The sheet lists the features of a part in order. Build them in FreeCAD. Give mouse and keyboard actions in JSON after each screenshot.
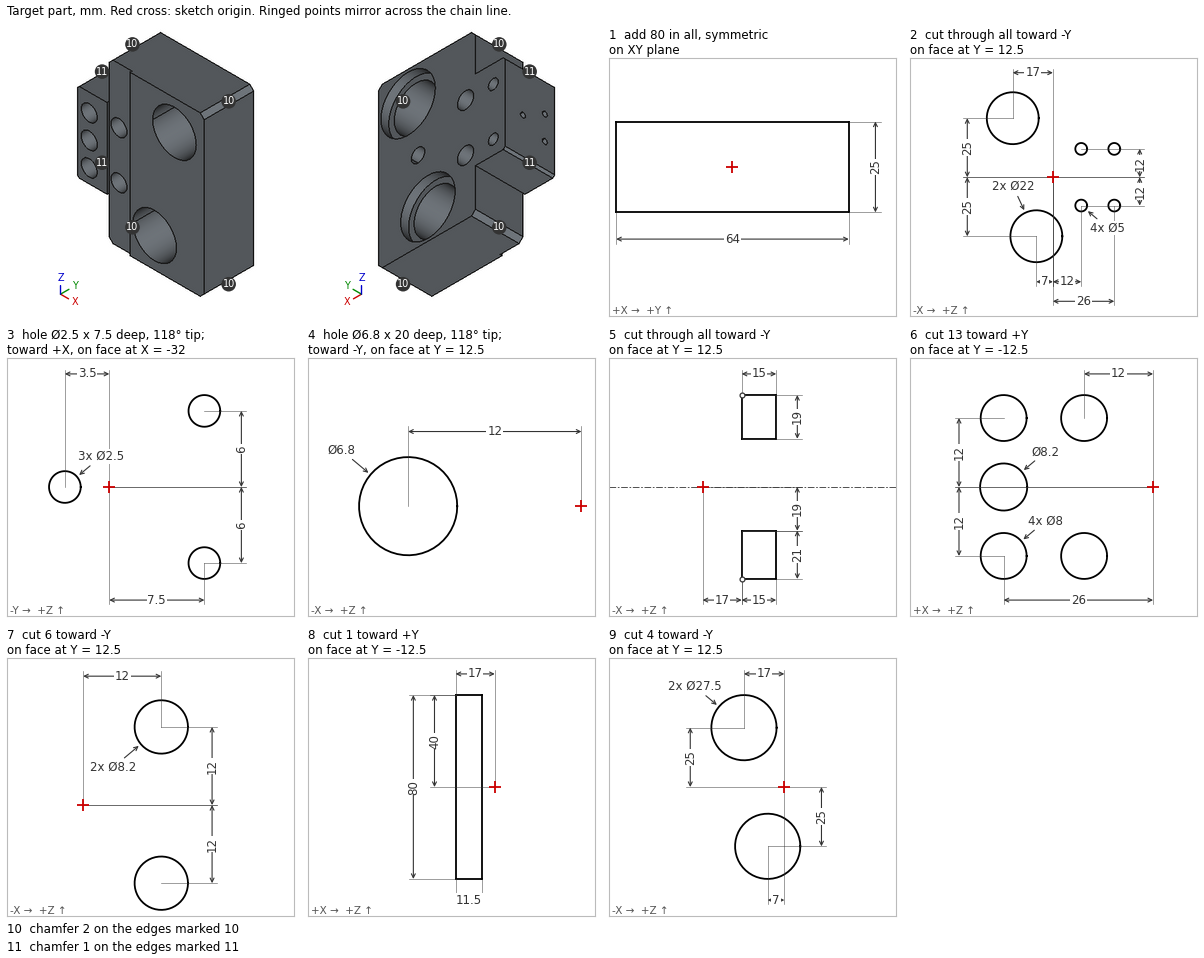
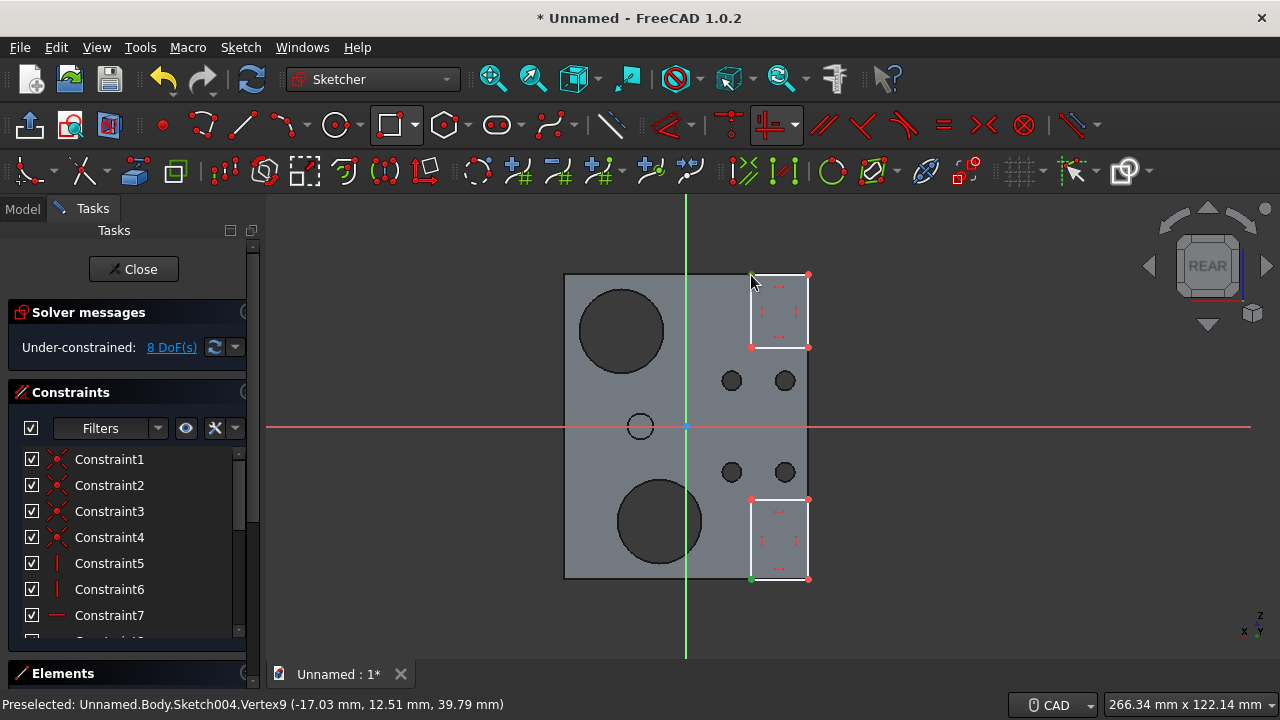
{"action": "left_click", "coordinate": [353, 427]}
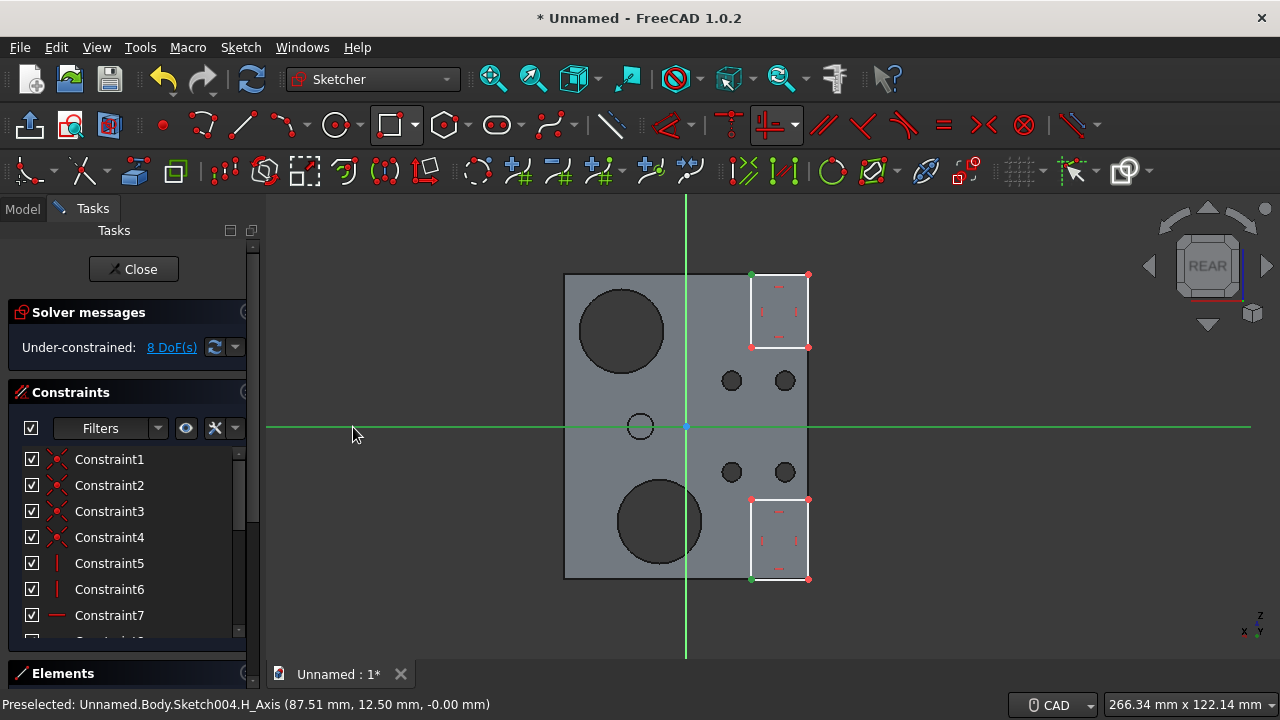
{"action": "left_click", "coordinate": [984, 126]}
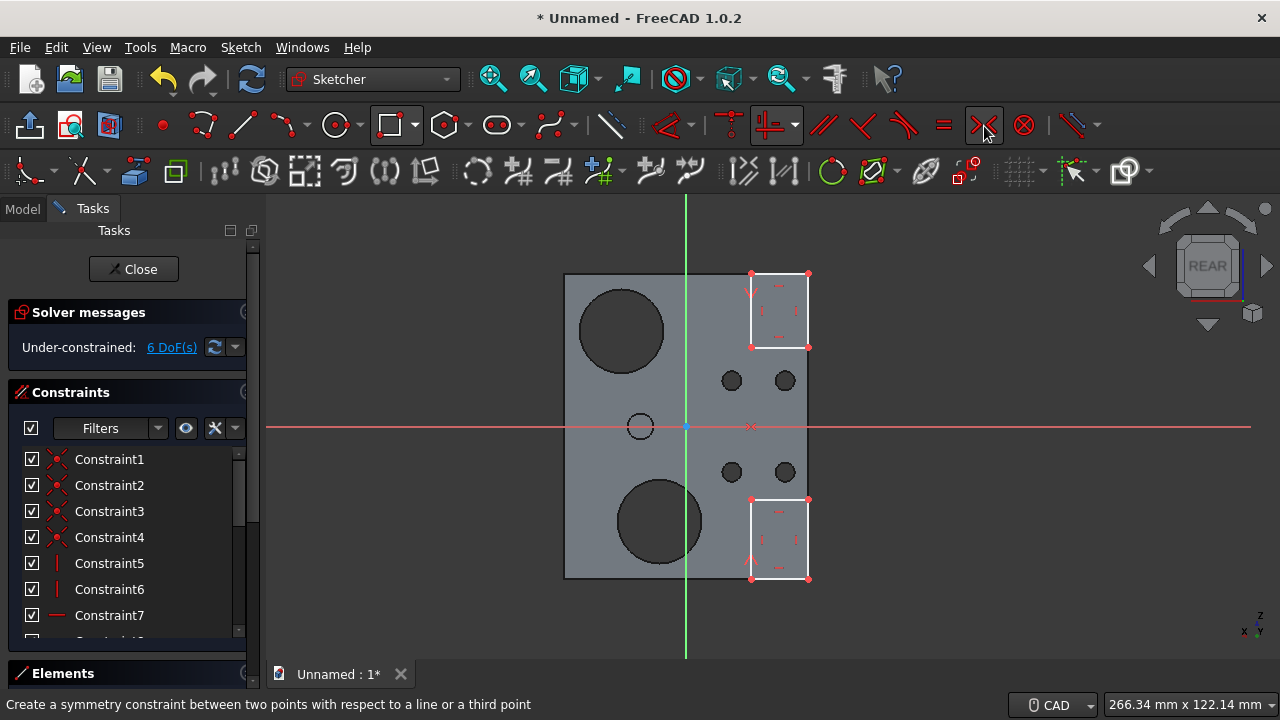
{"action": "left_click", "coordinate": [666, 126]}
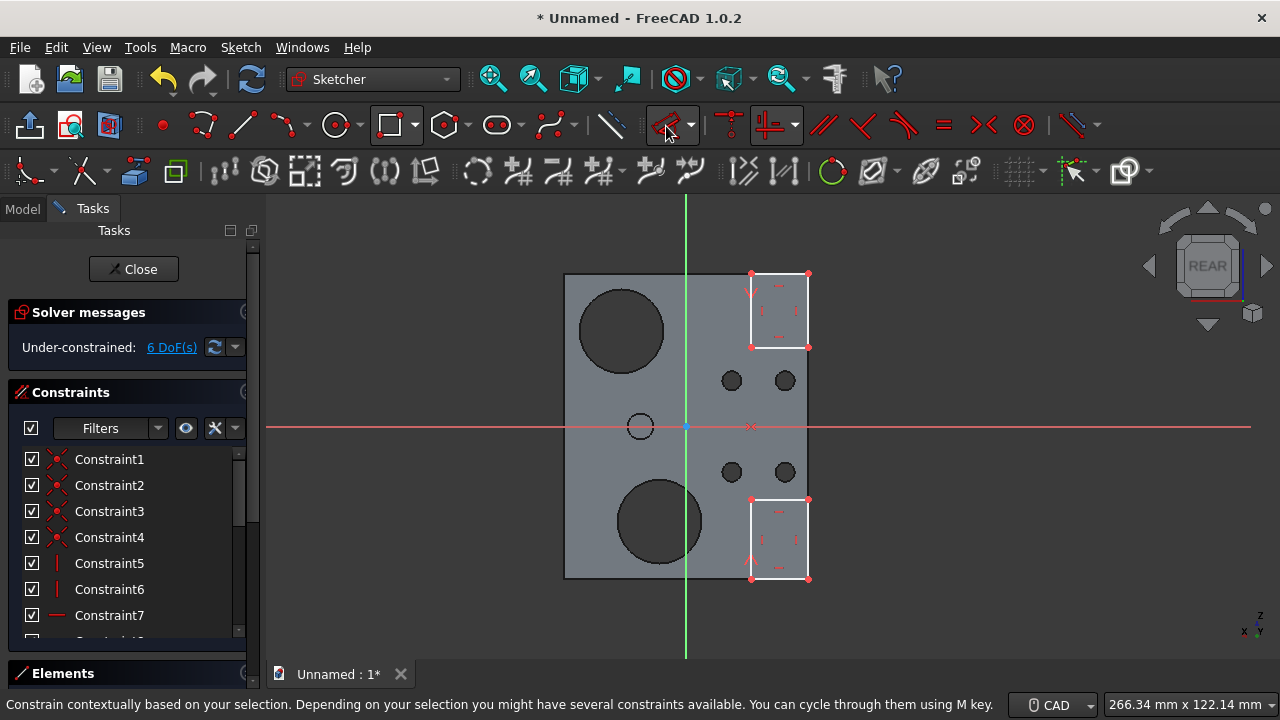
{"action": "left_click", "coordinate": [751, 524]}
{"action": "left_click", "coordinate": [785, 540]}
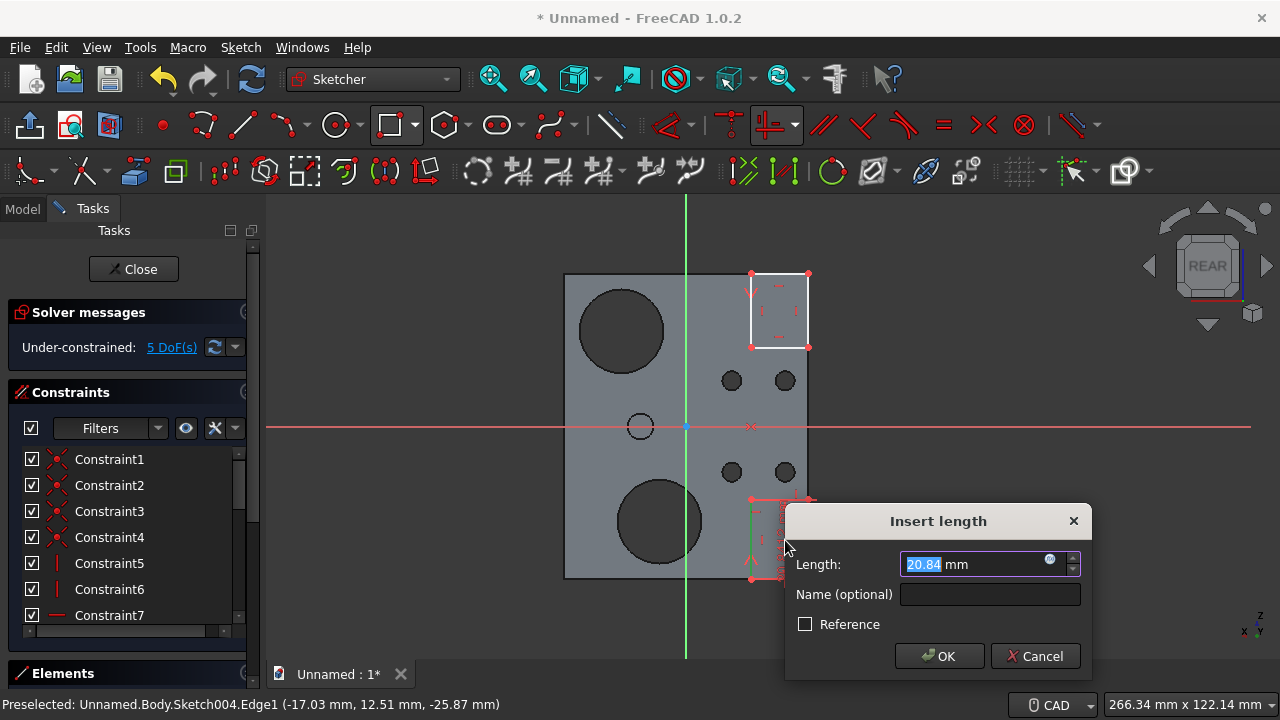
{"action": "type", "text": "21"}
{"action": "key", "text": "Return"}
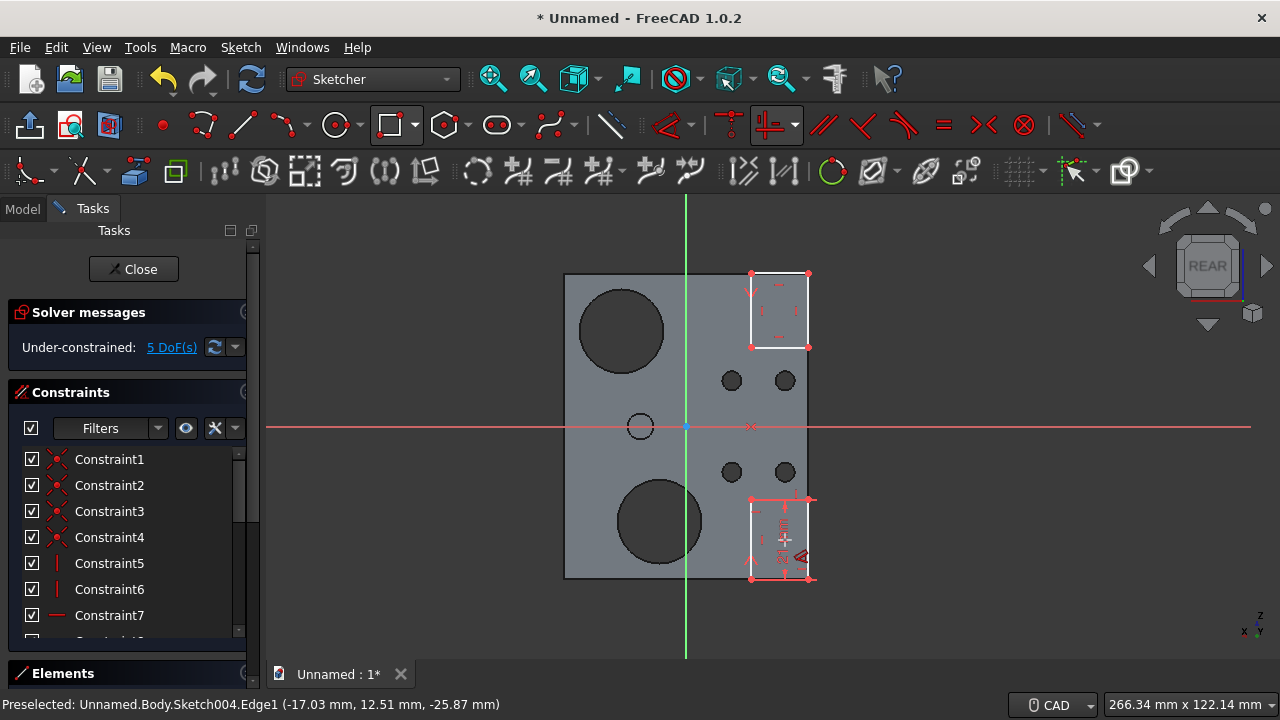
{"action": "left_click", "coordinate": [768, 580]}
{"action": "left_click", "coordinate": [779, 614]}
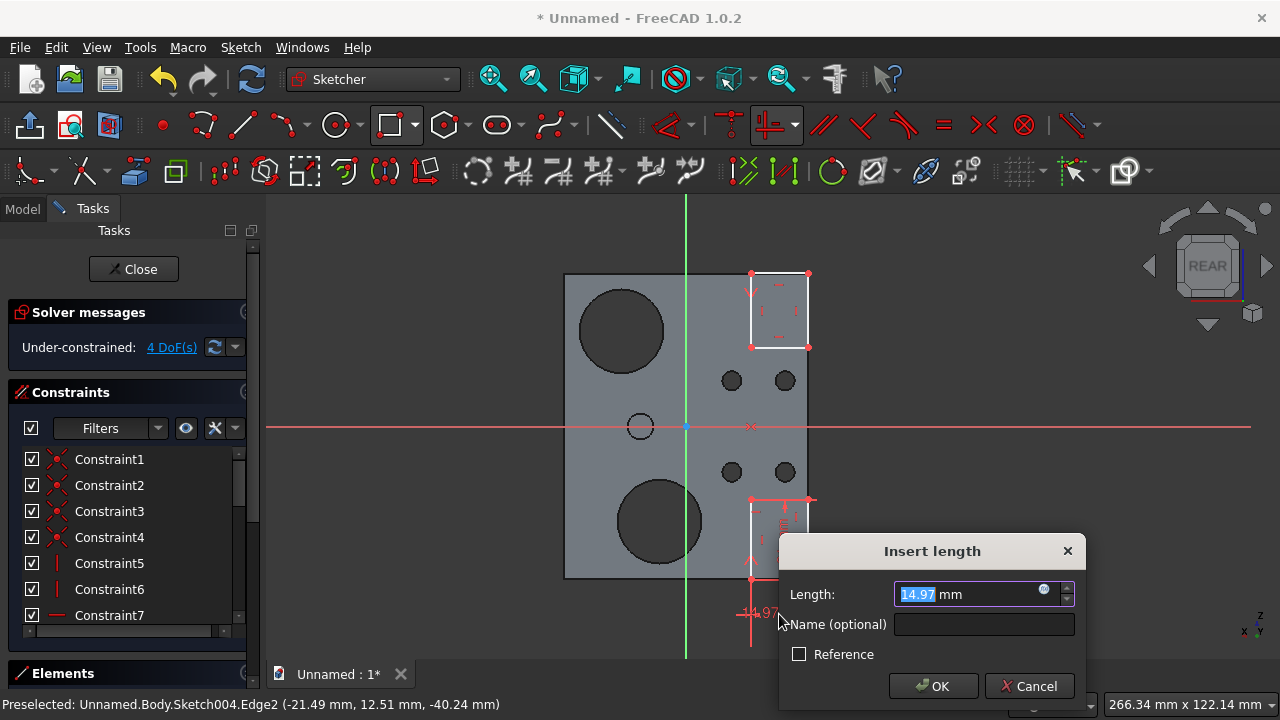
{"action": "type", "text": "15"}
{"action": "key", "text": "Return"}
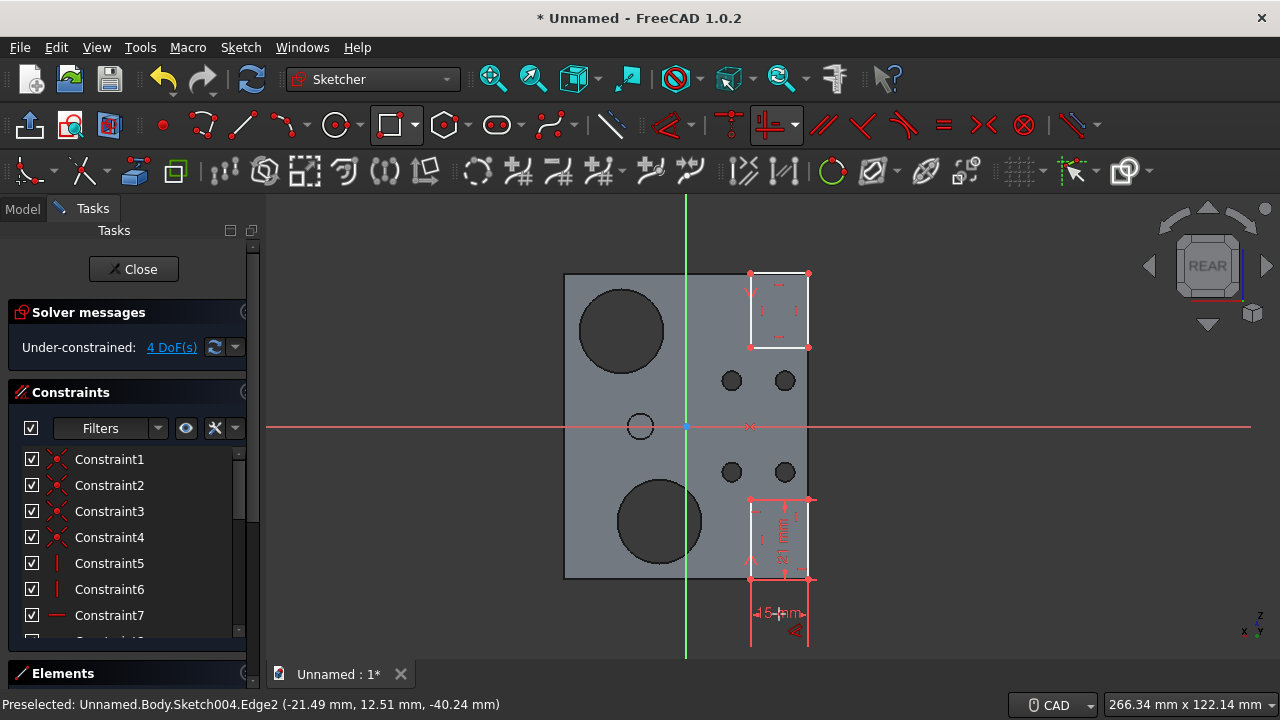
{"action": "left_click", "coordinate": [751, 296]}
{"action": "left_click", "coordinate": [785, 311]}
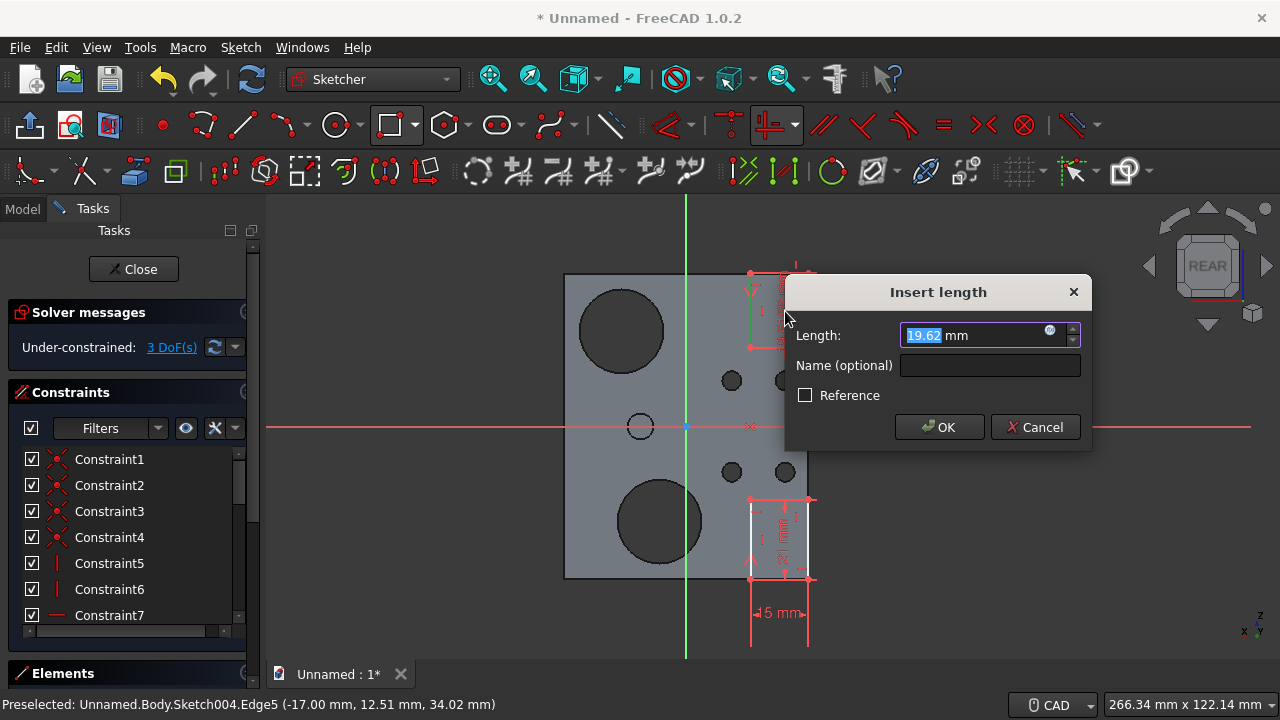
{"action": "type", "text": "19"}
{"action": "key", "text": "Return"}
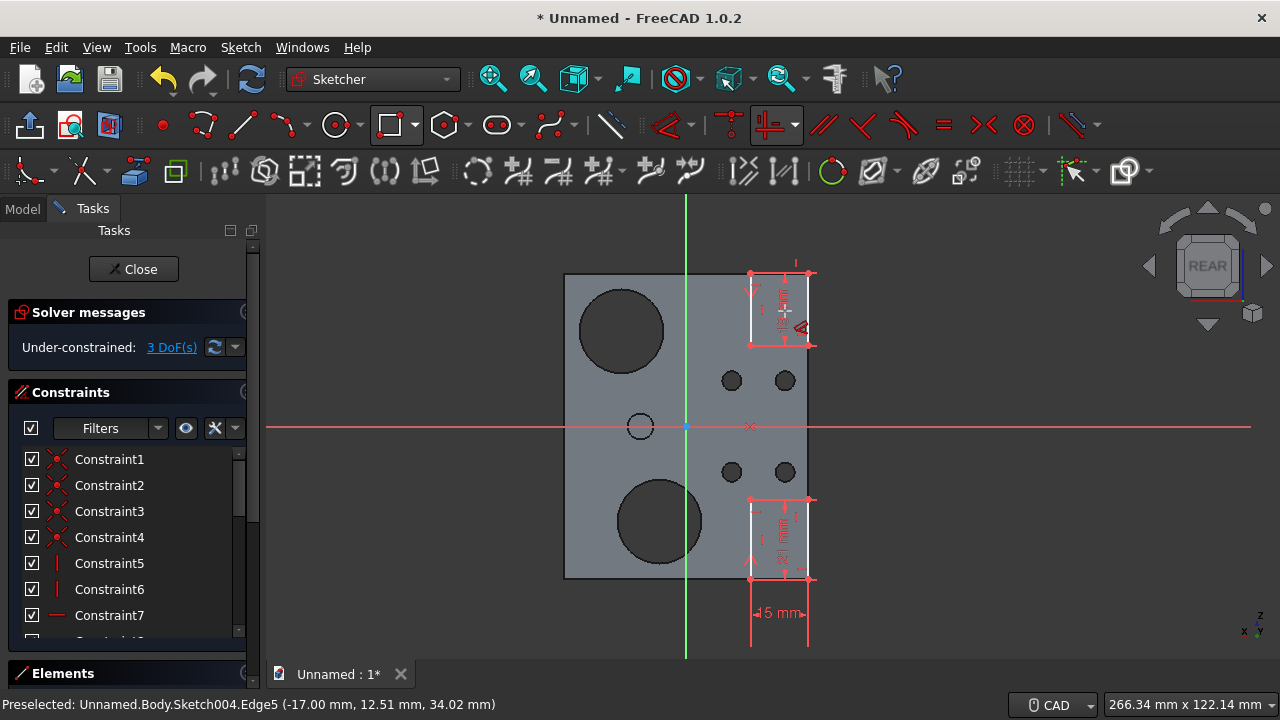
{"action": "left_click", "coordinate": [768, 346]}
{"action": "left_click", "coordinate": [779, 380]}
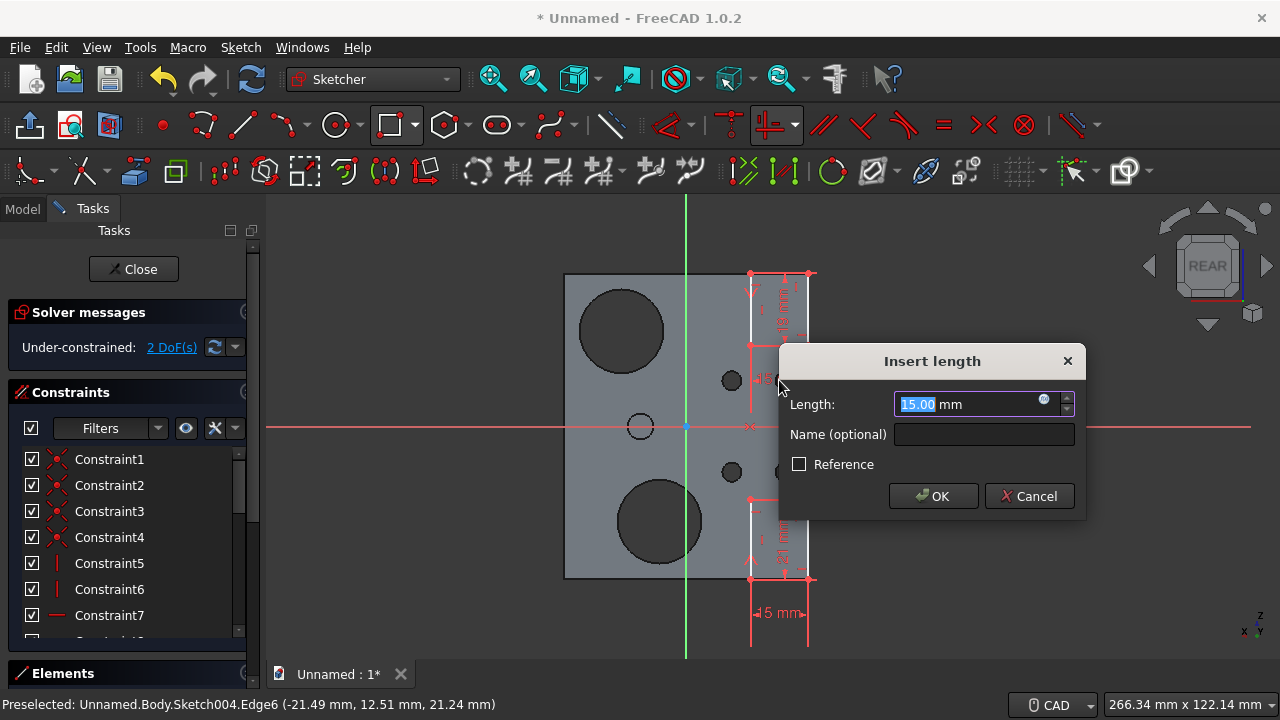
{"action": "type", "text": "15"}
{"action": "key", "text": "Return"}